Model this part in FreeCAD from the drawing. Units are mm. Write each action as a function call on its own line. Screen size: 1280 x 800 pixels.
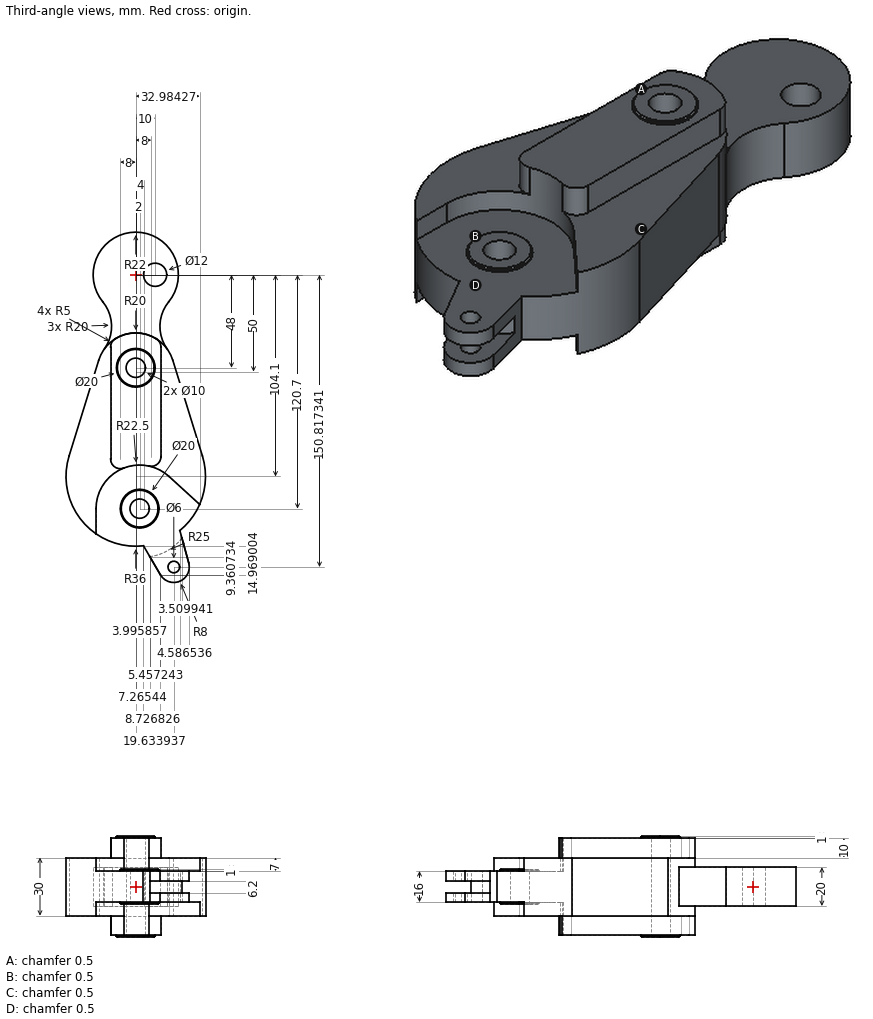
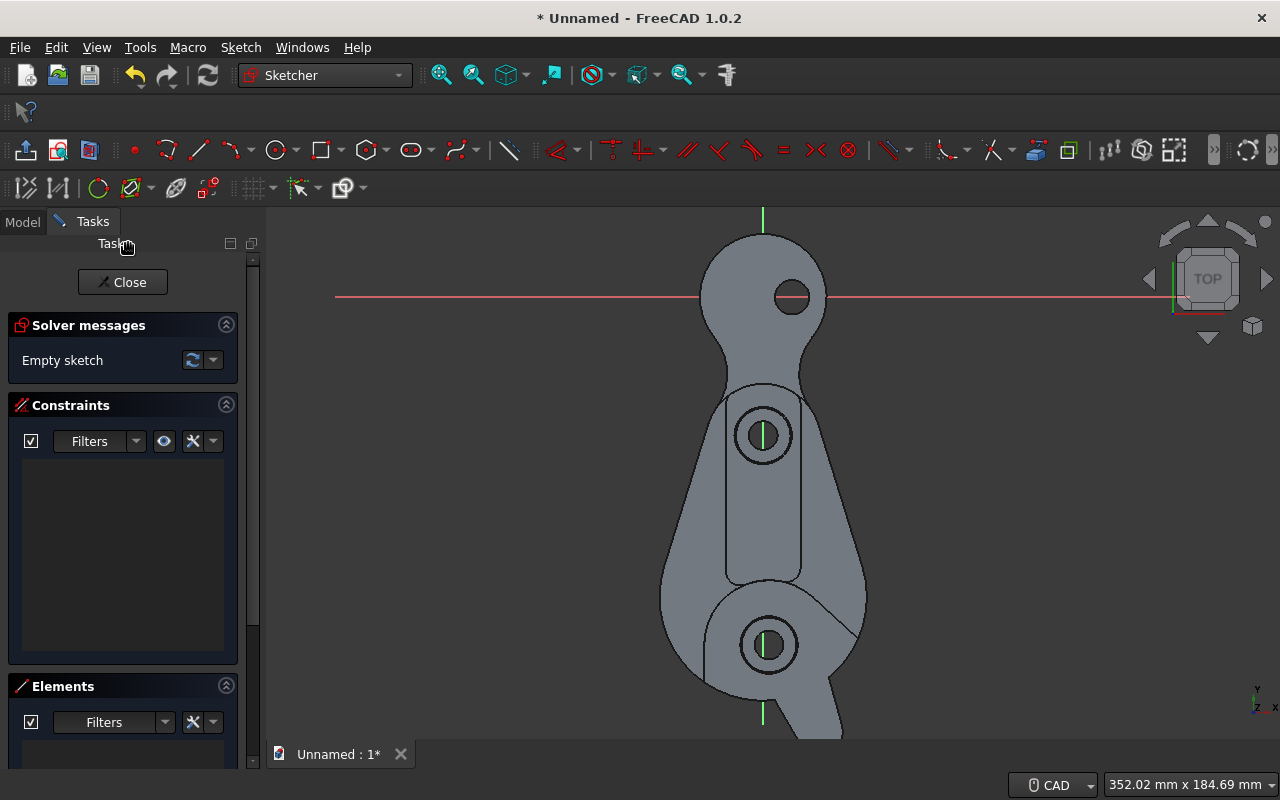
click(90, 150)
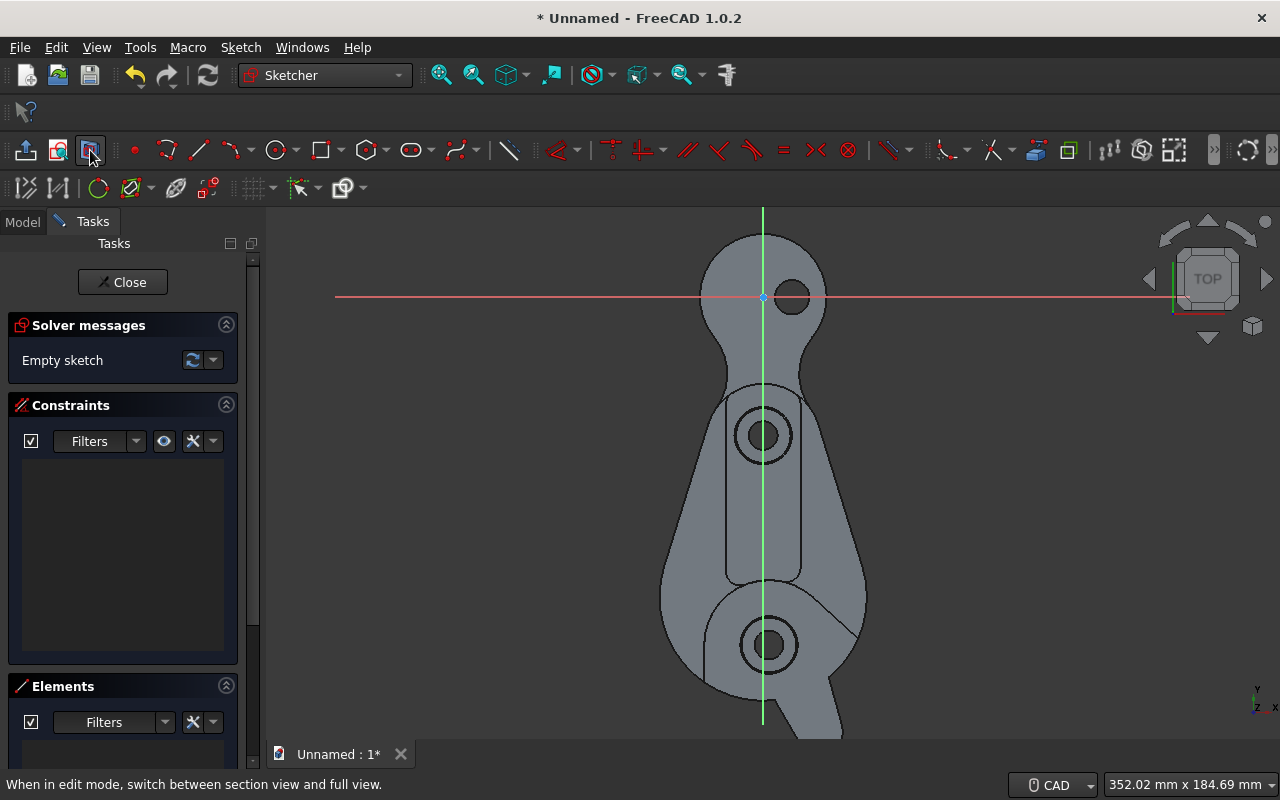
scroll(704, 473, down, 5)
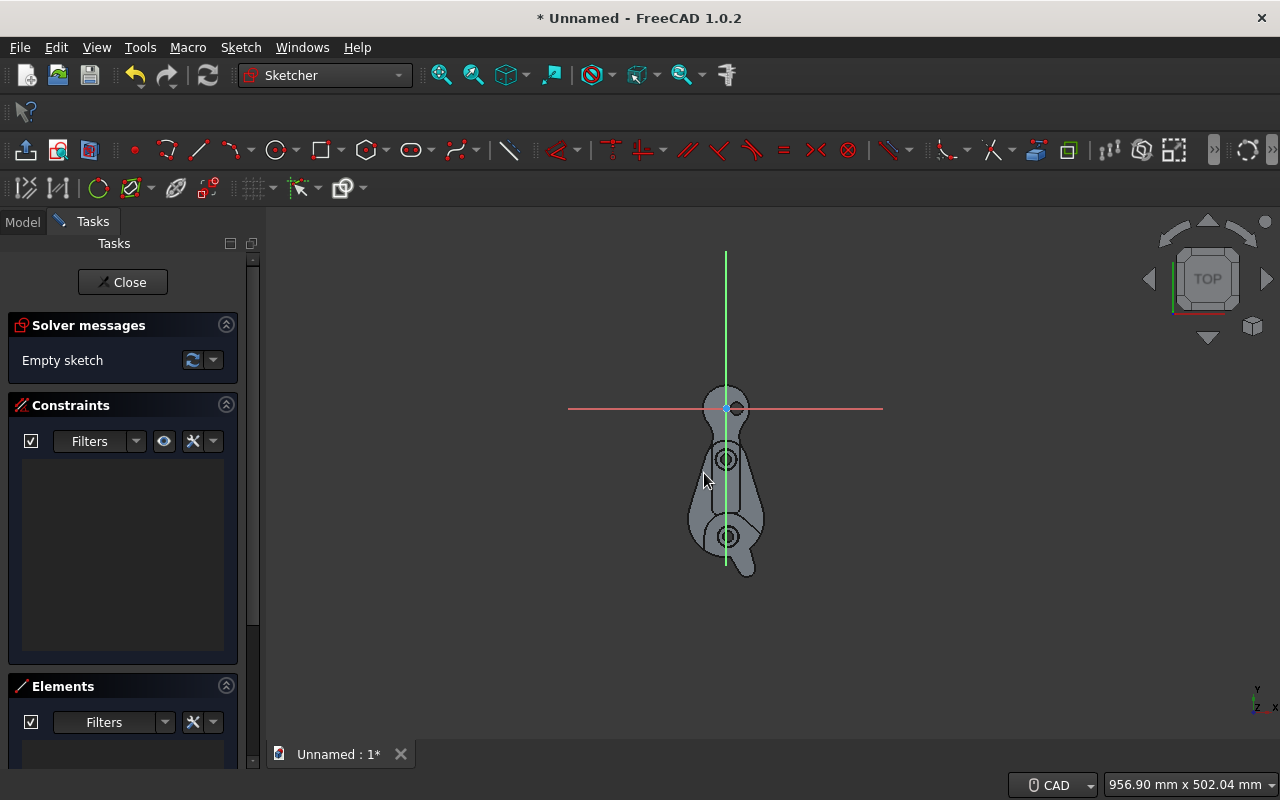
scroll(748, 572, up, 13)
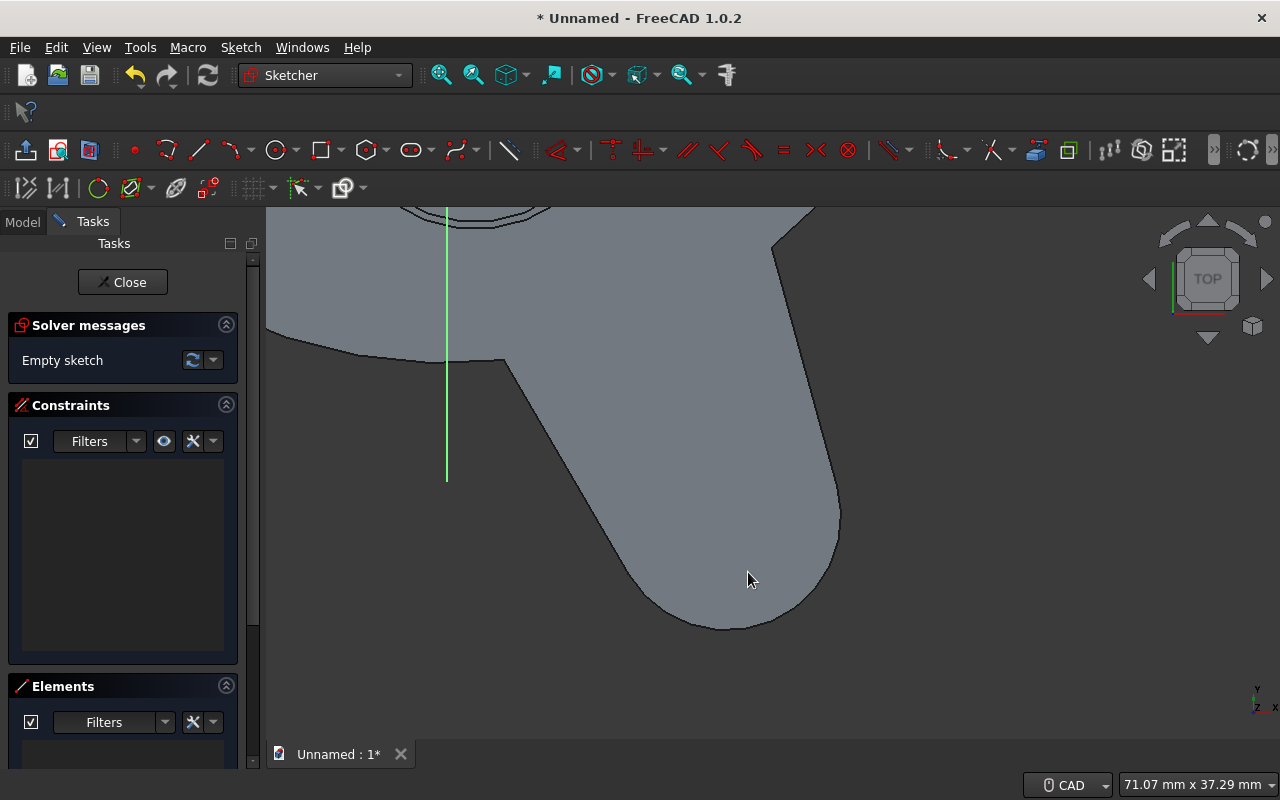
click(200, 150)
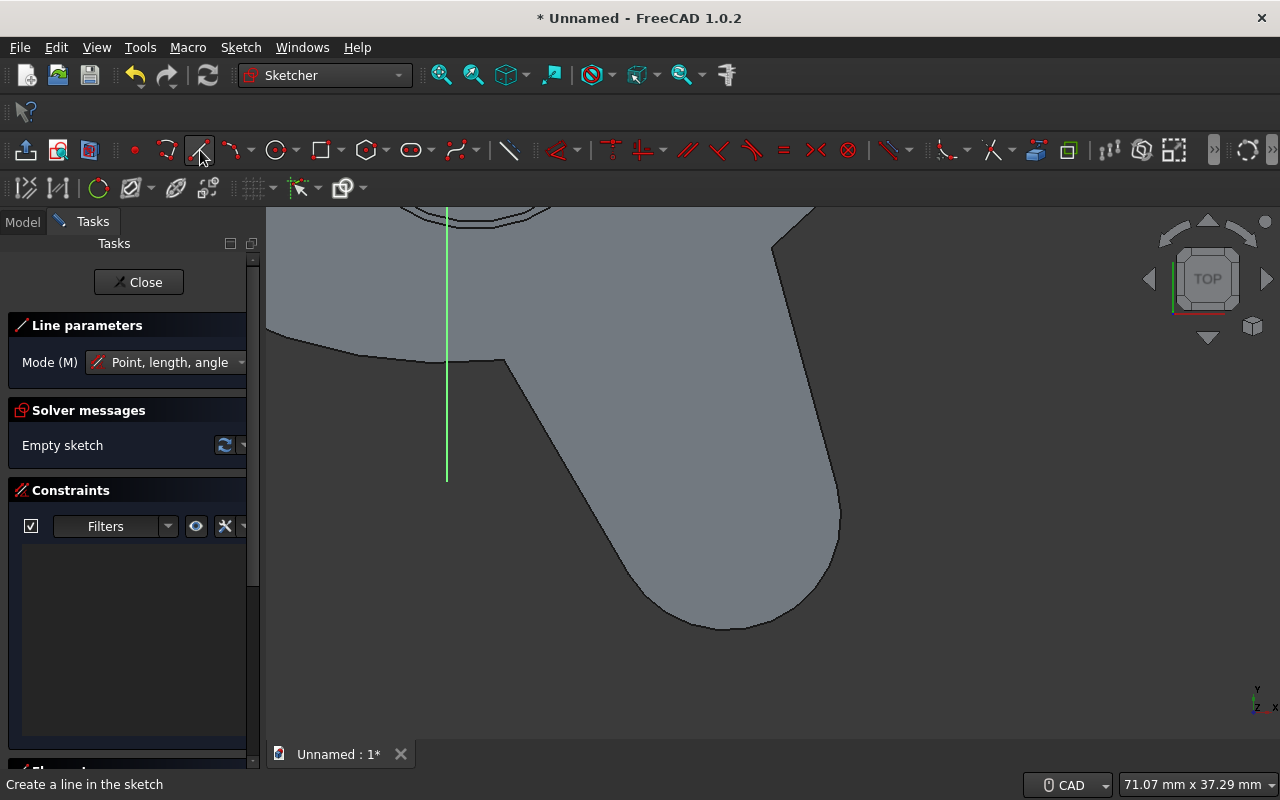
click(837, 486)
click(787, 304)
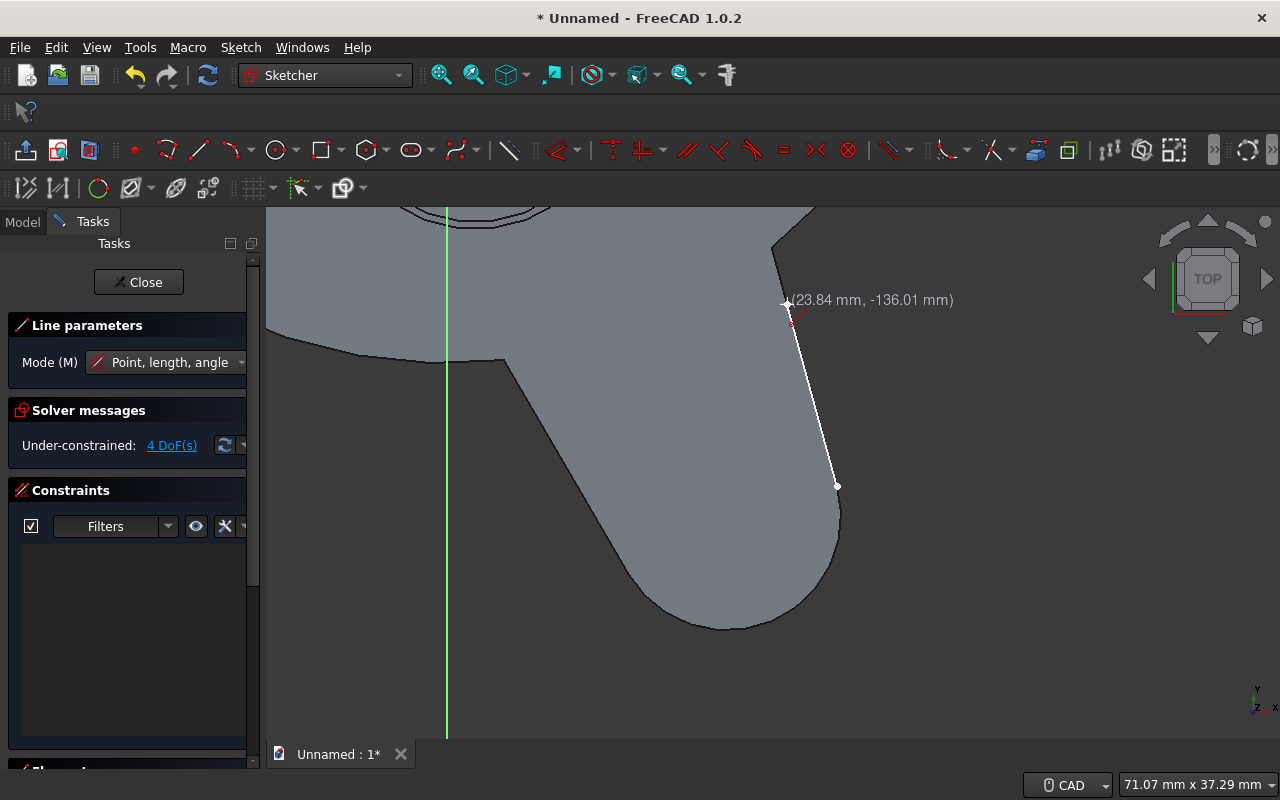
click(550, 440)
click(628, 574)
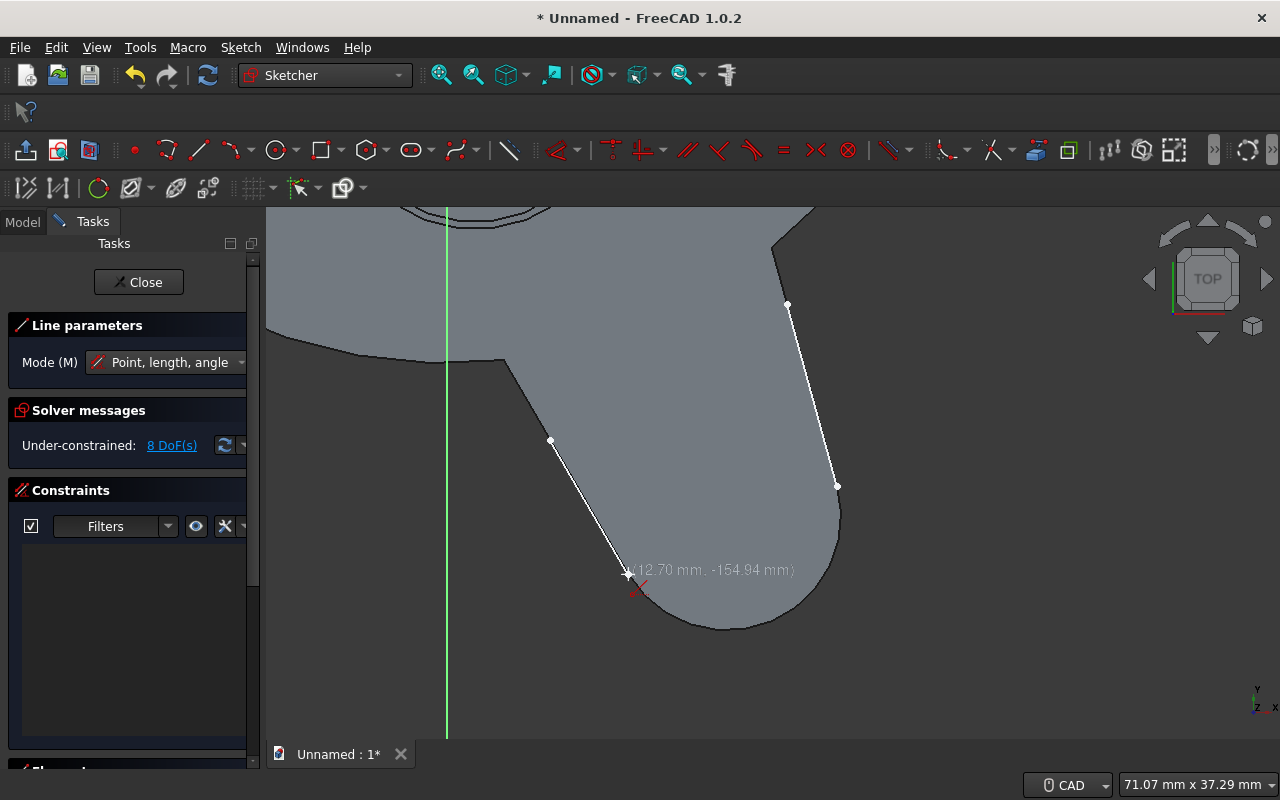
click(232, 150)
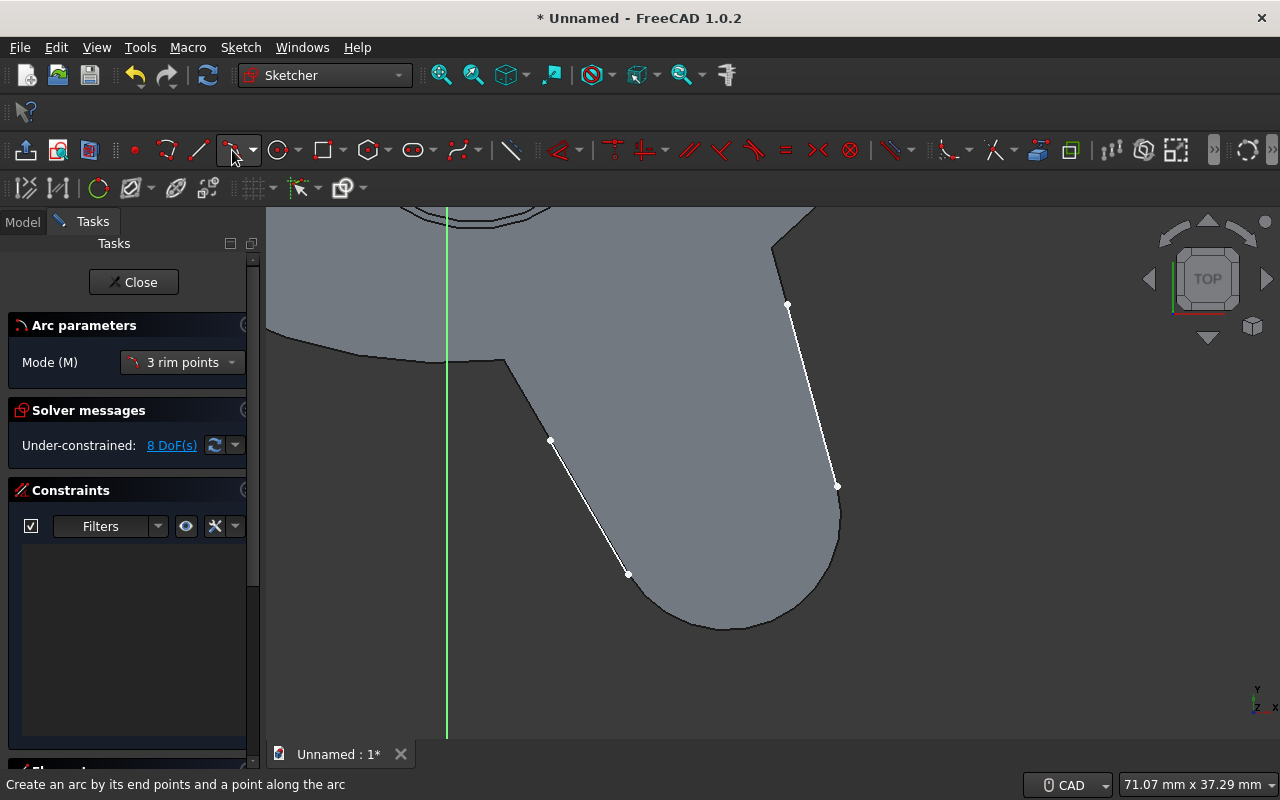
click(787, 305)
click(550, 441)
click(682, 395)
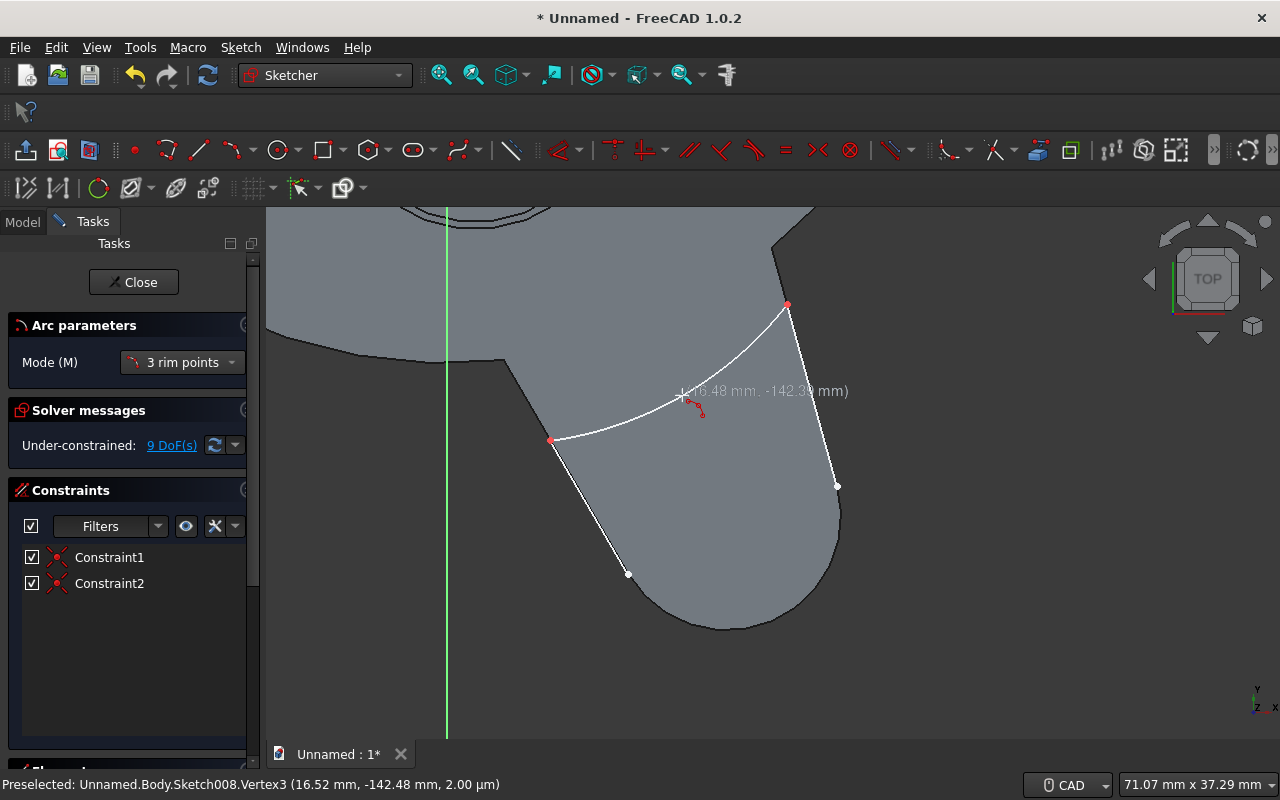
click(628, 575)
click(837, 487)
click(771, 621)
key(Escape)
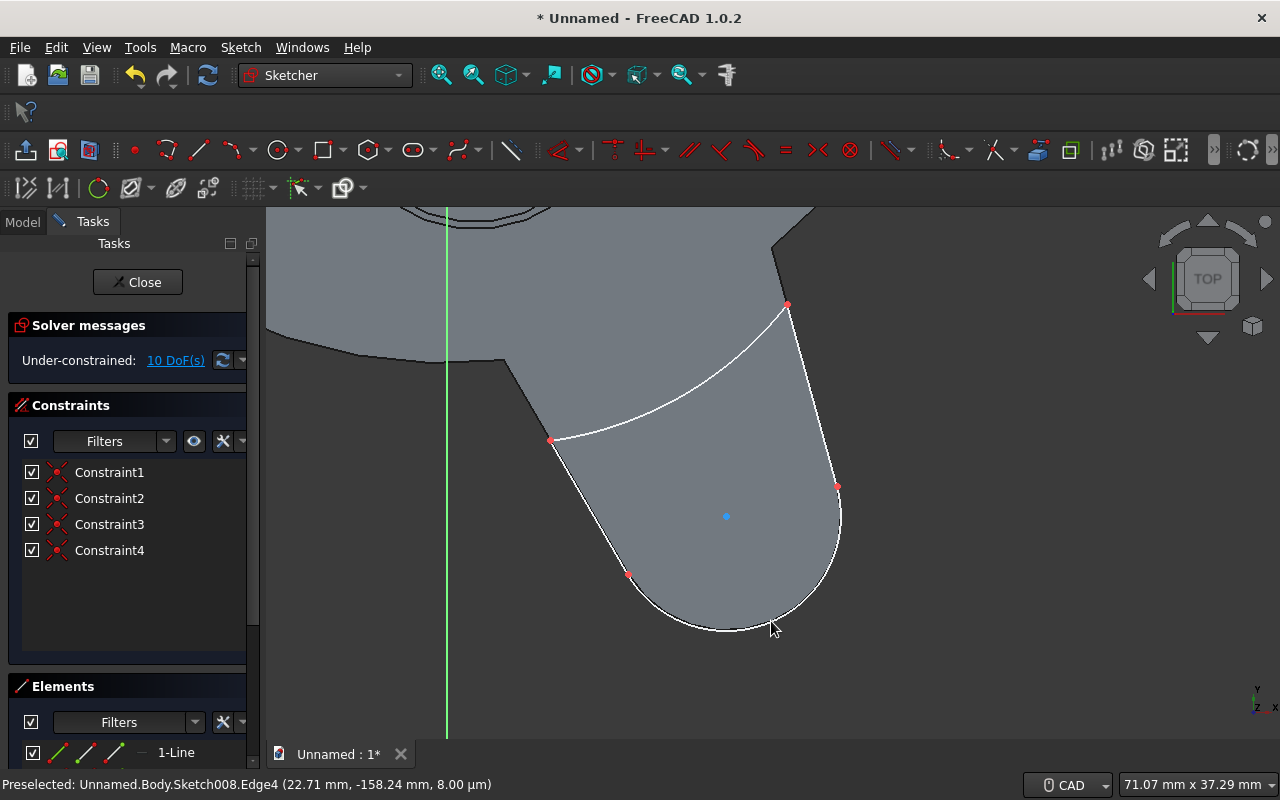
click(822, 432)